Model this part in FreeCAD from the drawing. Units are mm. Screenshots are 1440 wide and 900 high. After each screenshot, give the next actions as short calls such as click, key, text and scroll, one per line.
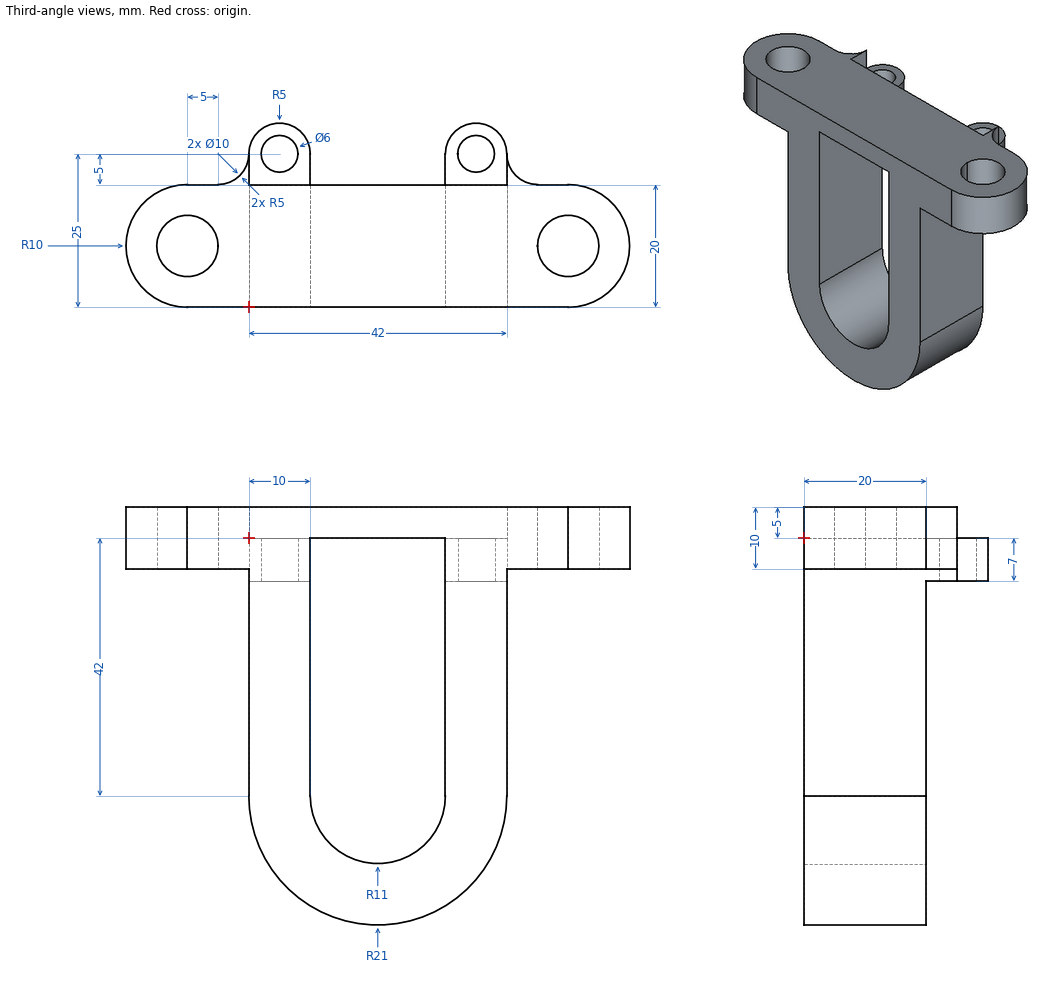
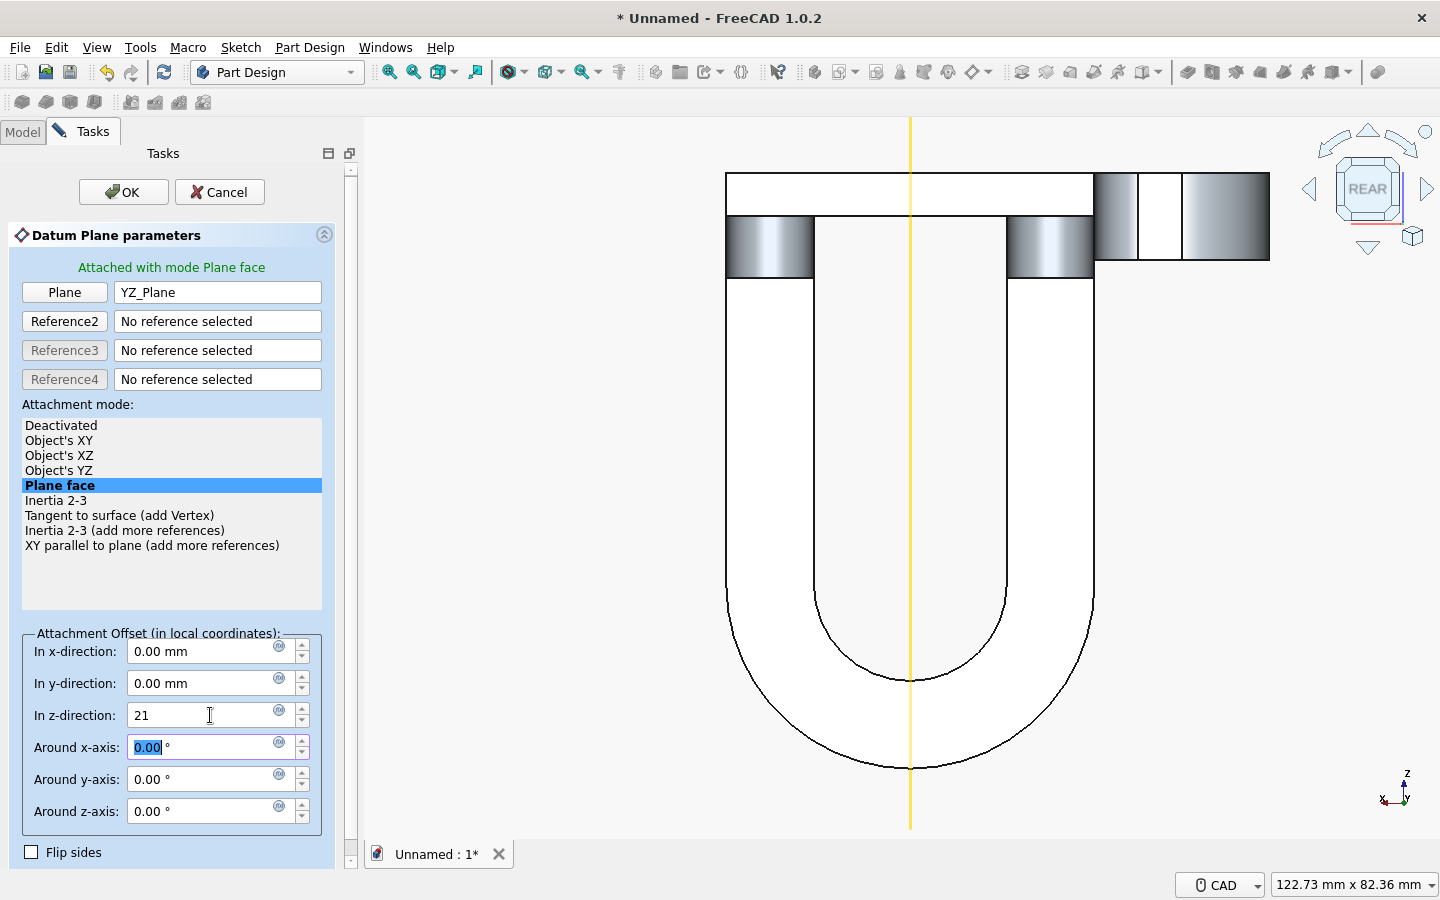
click(124, 192)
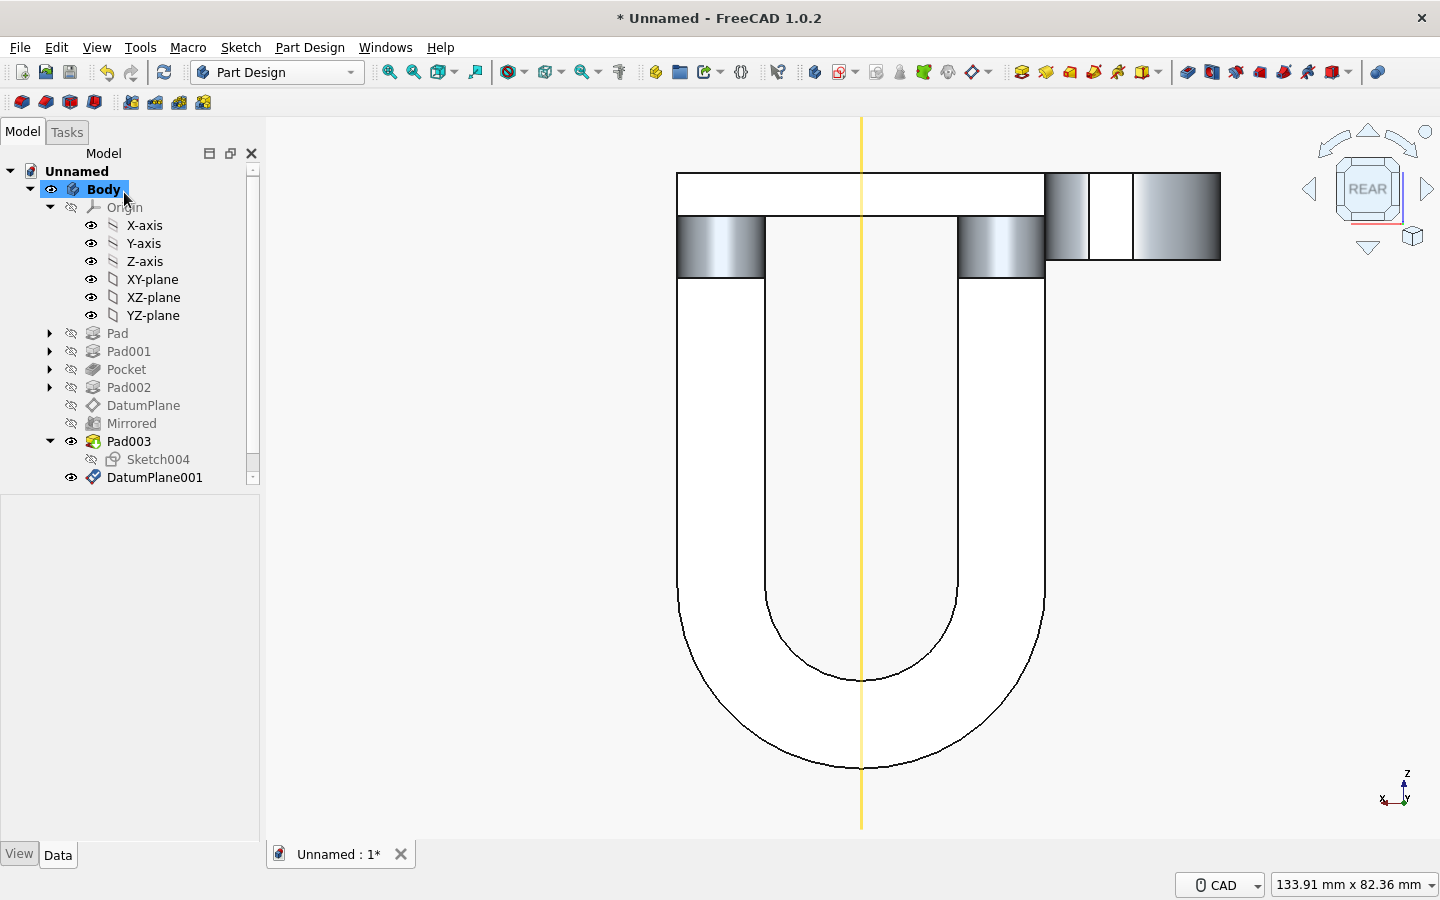
click(116, 441)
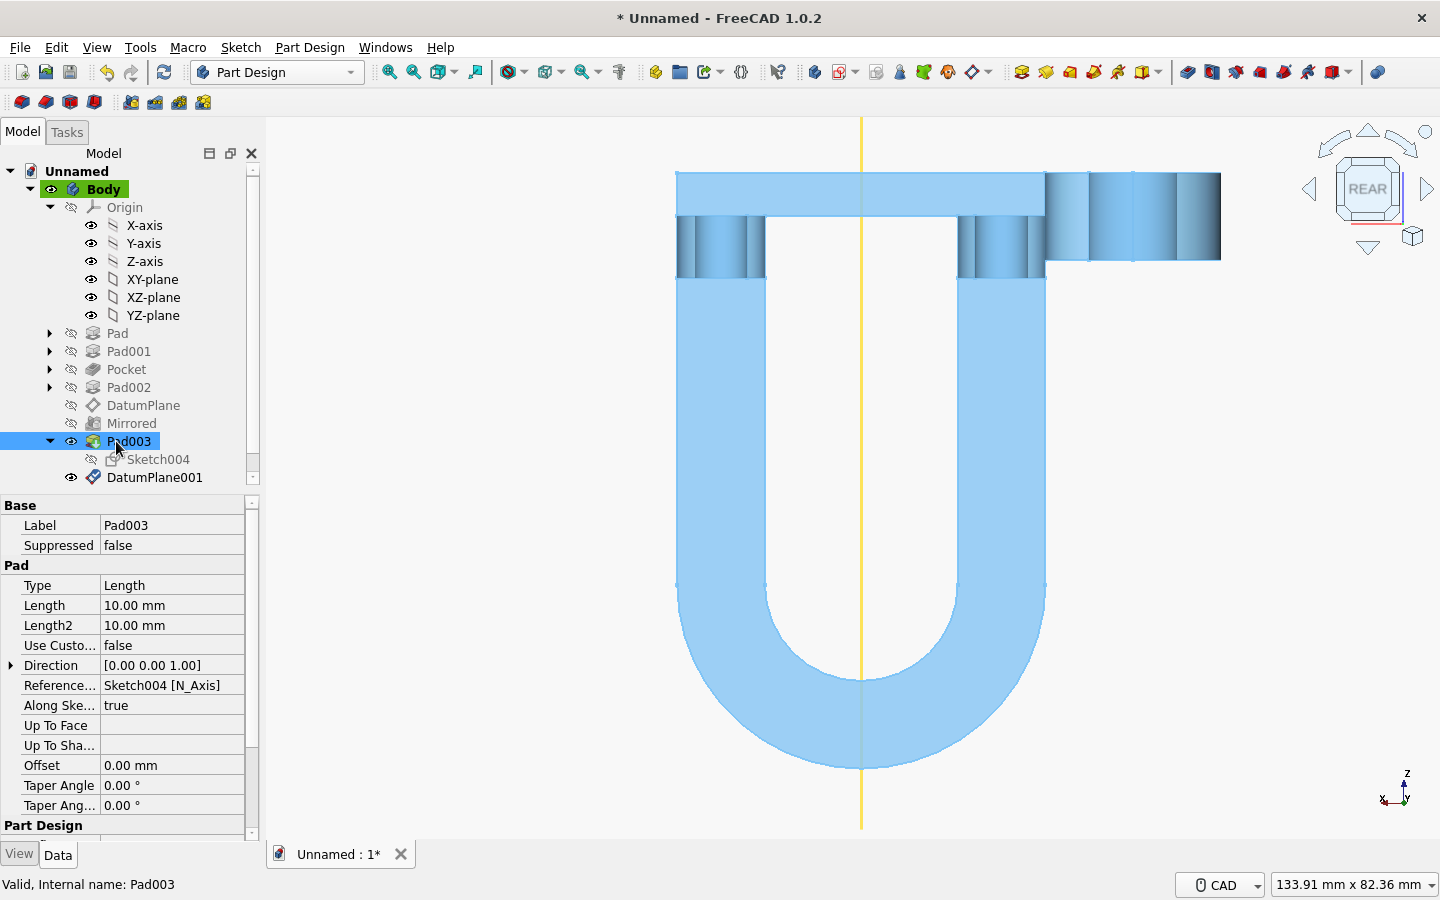
click(132, 102)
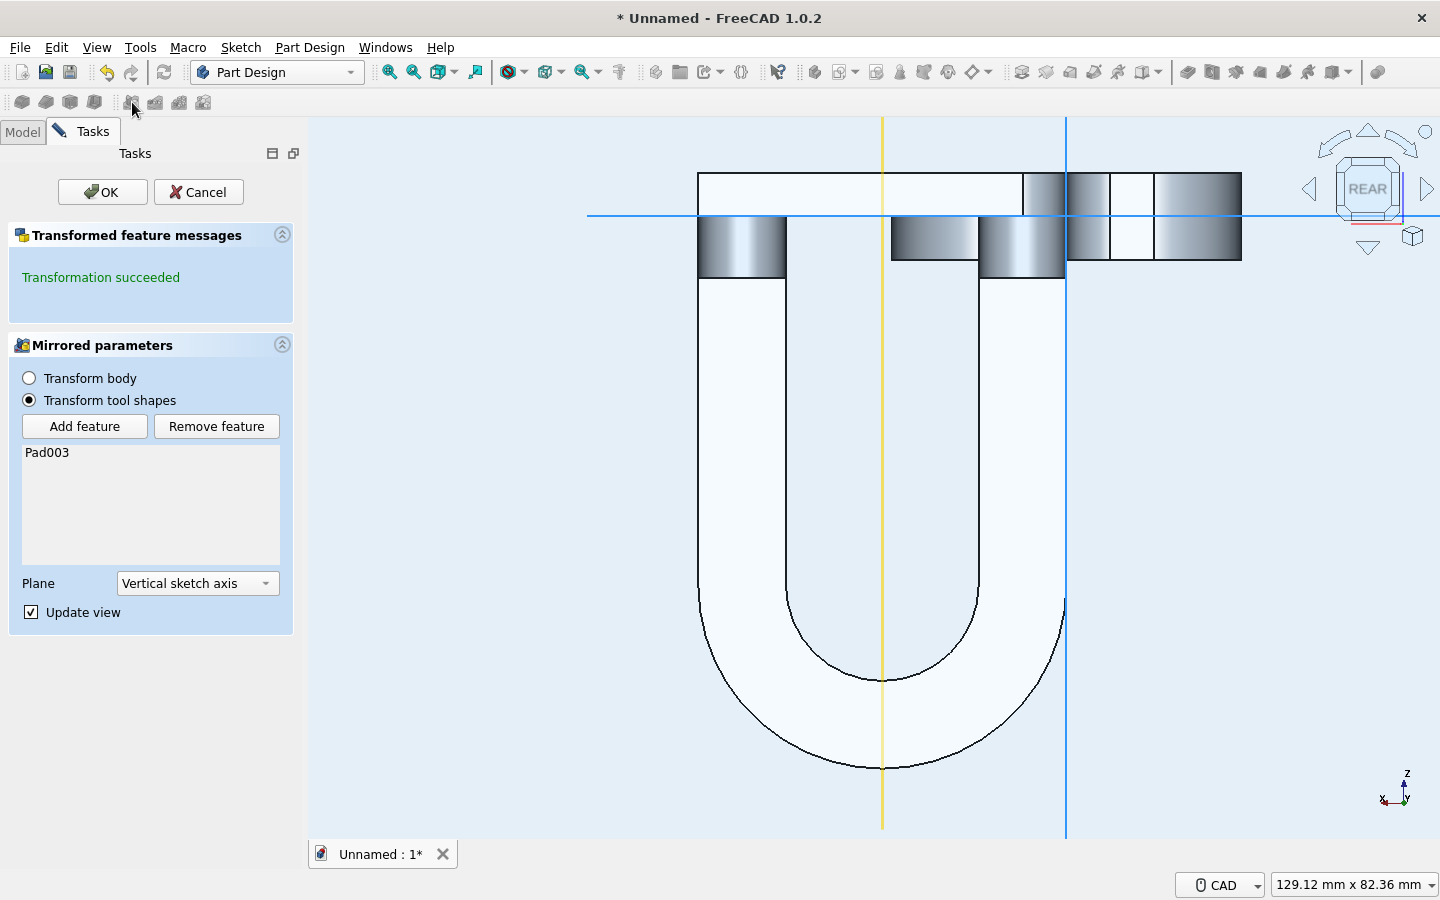
click(198, 584)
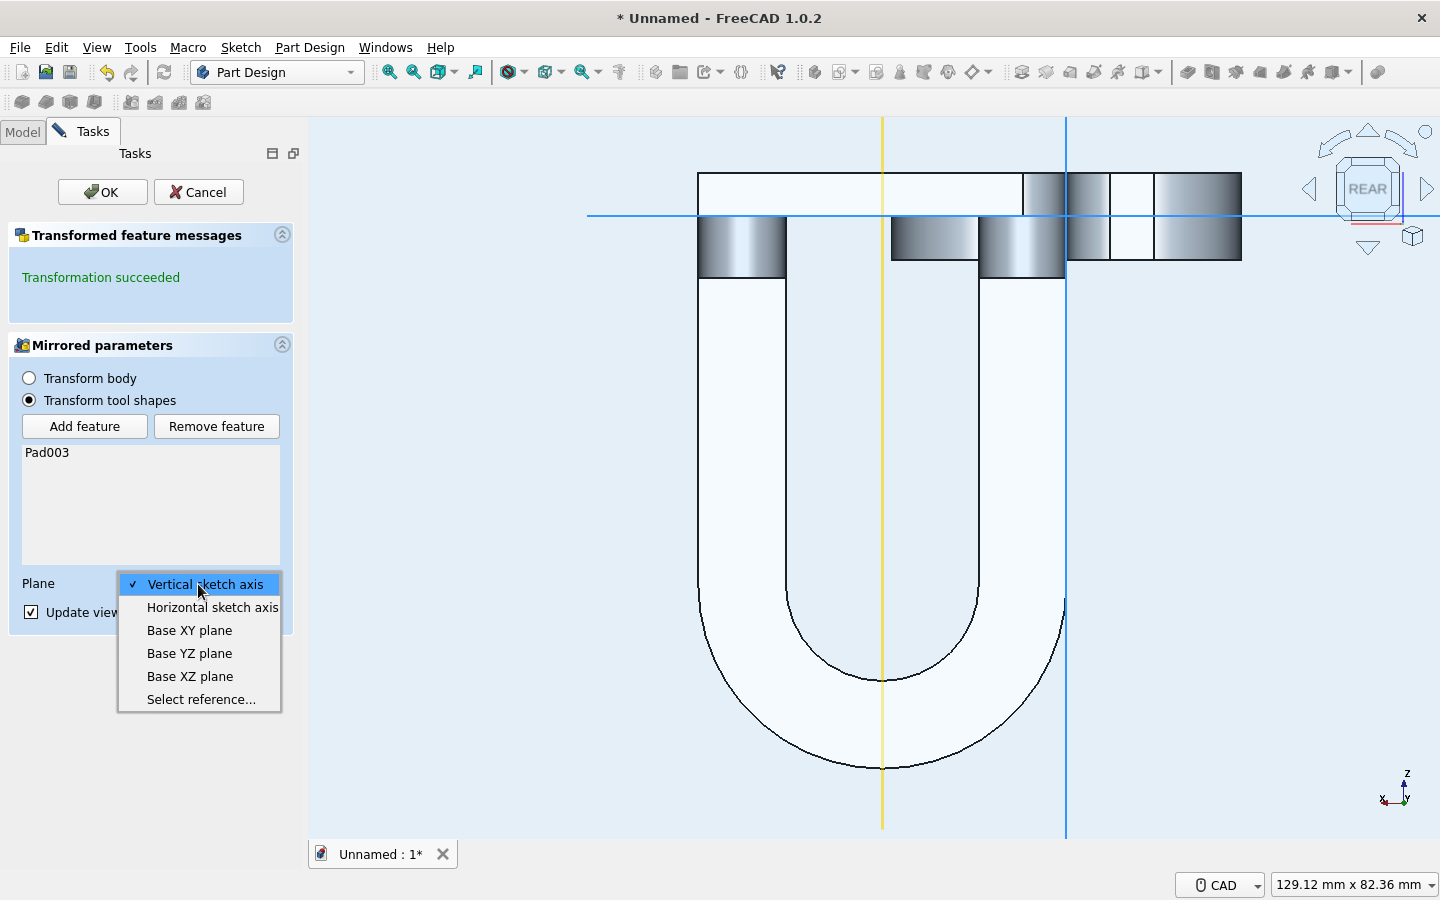
click(198, 700)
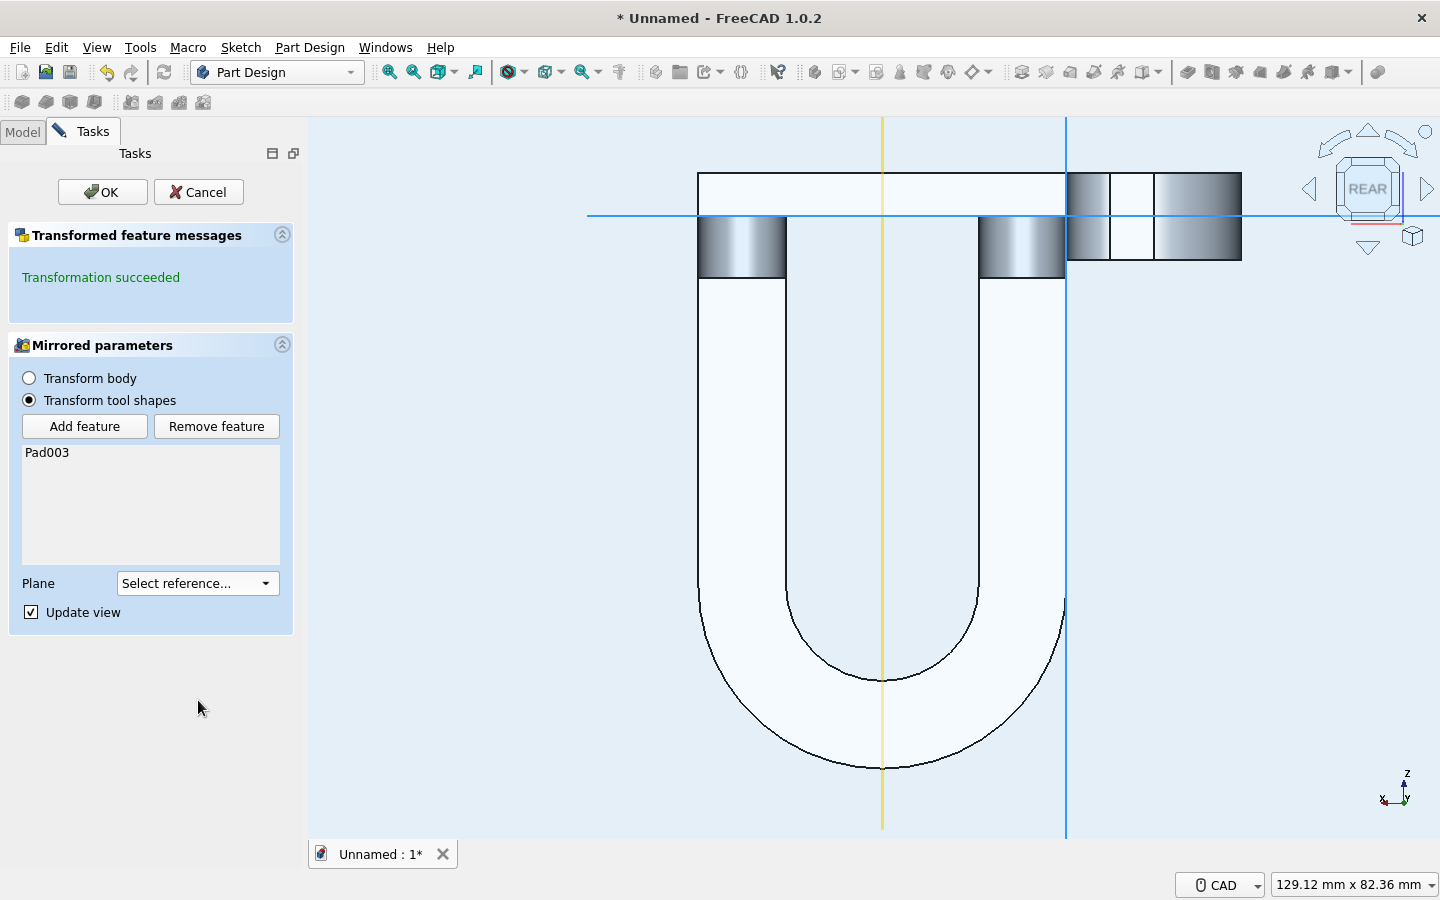
click(23, 131)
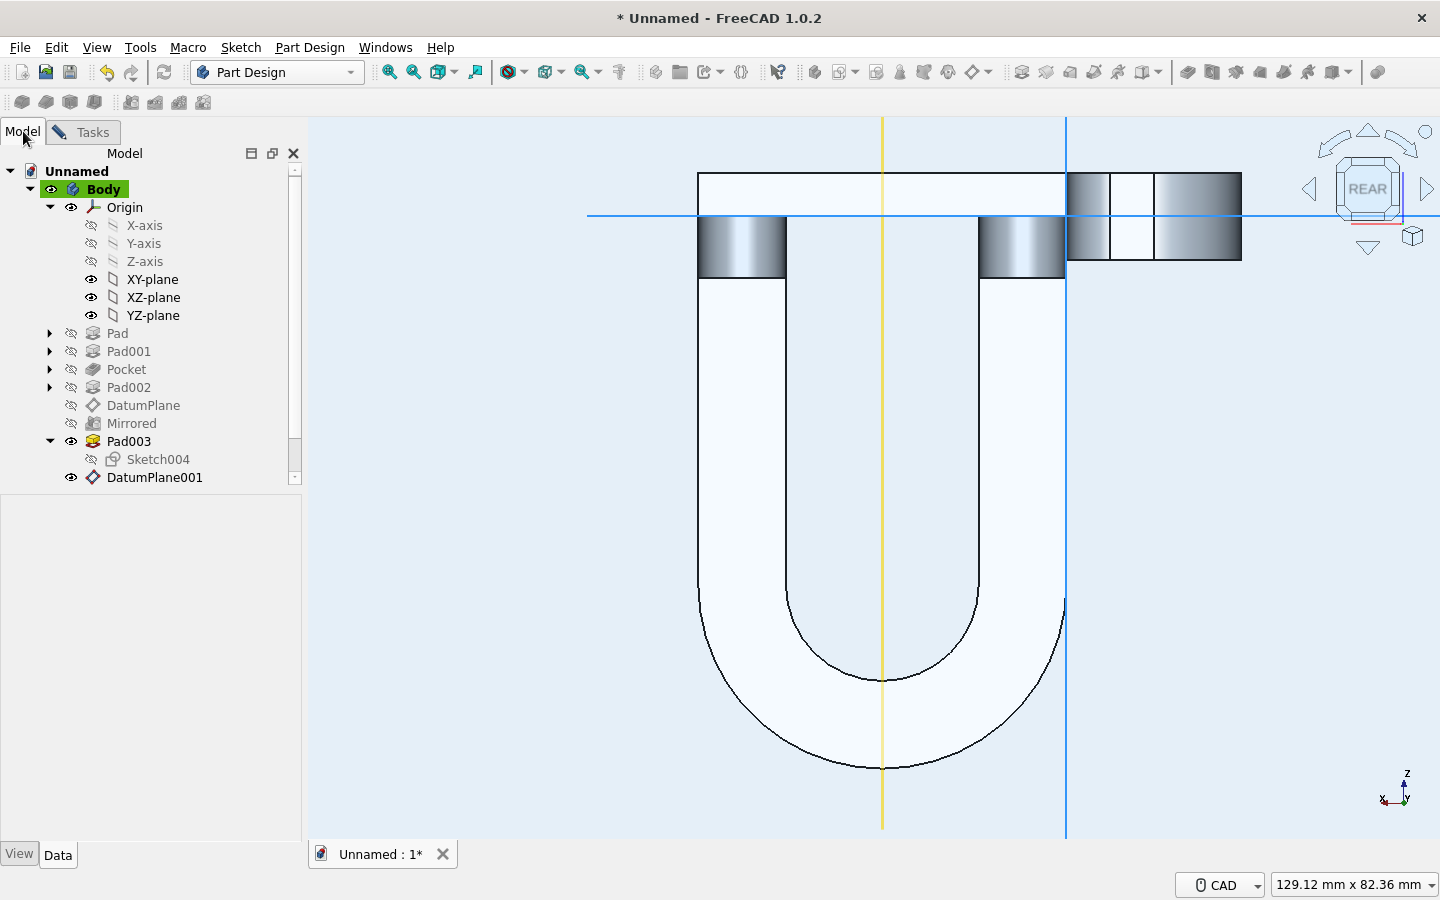
click(116, 477)